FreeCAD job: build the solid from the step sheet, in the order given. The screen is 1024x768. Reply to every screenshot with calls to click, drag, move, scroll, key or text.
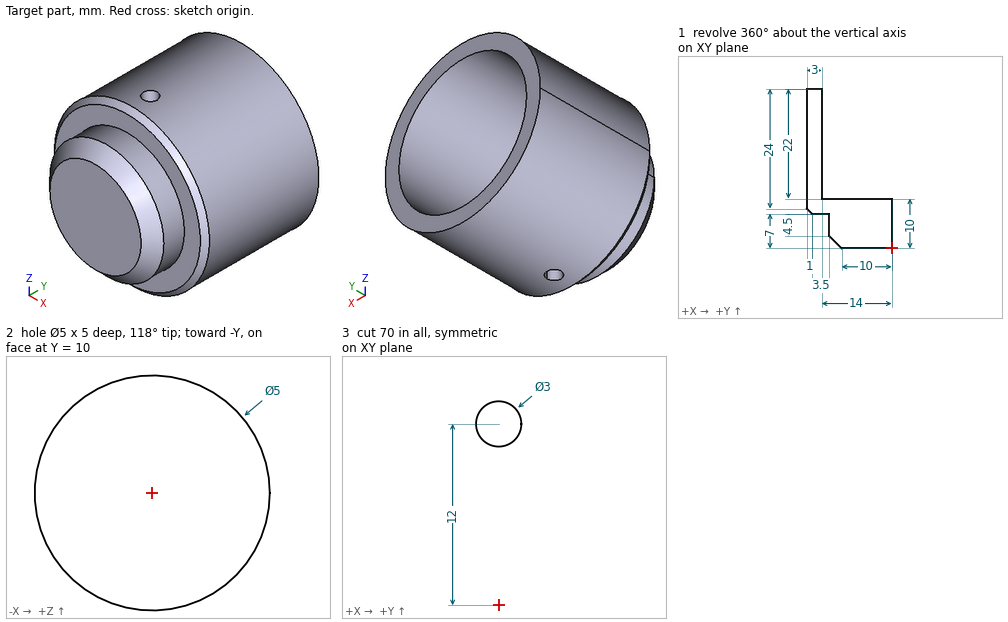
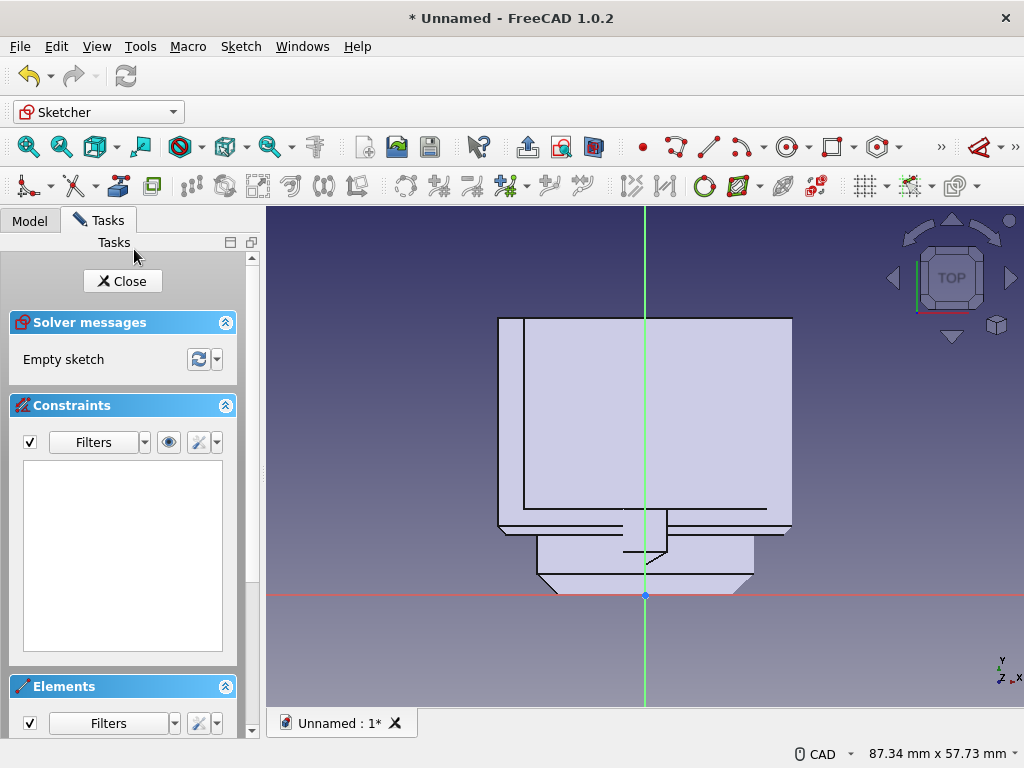
scroll(652, 495, up, 12)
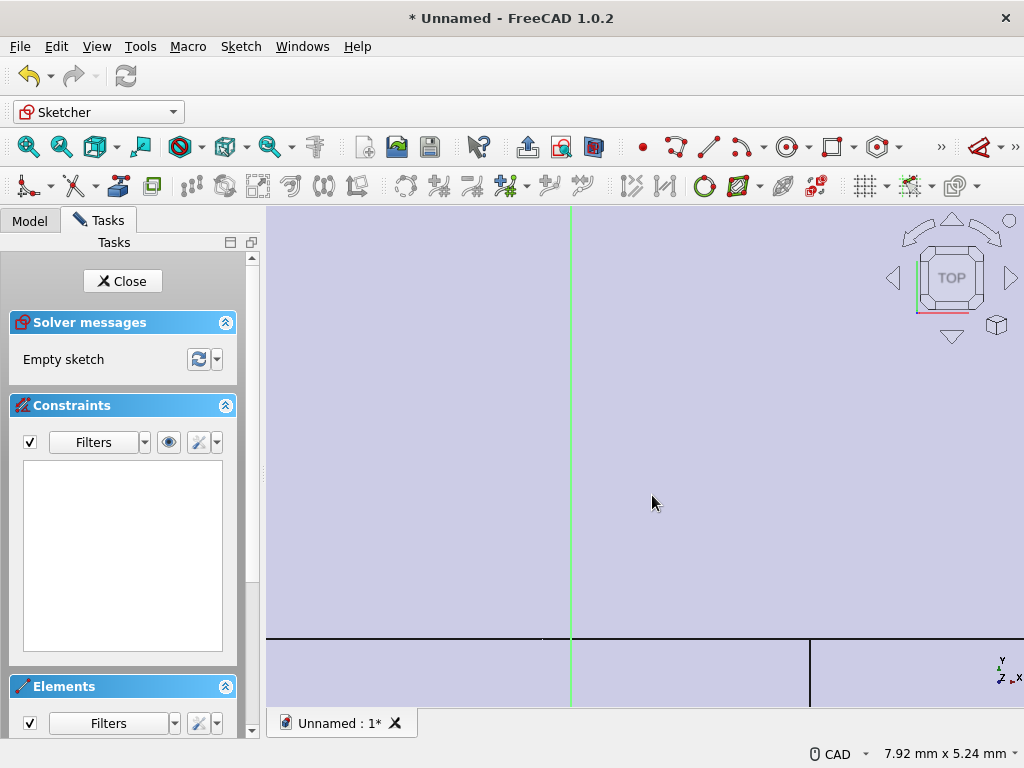
key(g)
key(c)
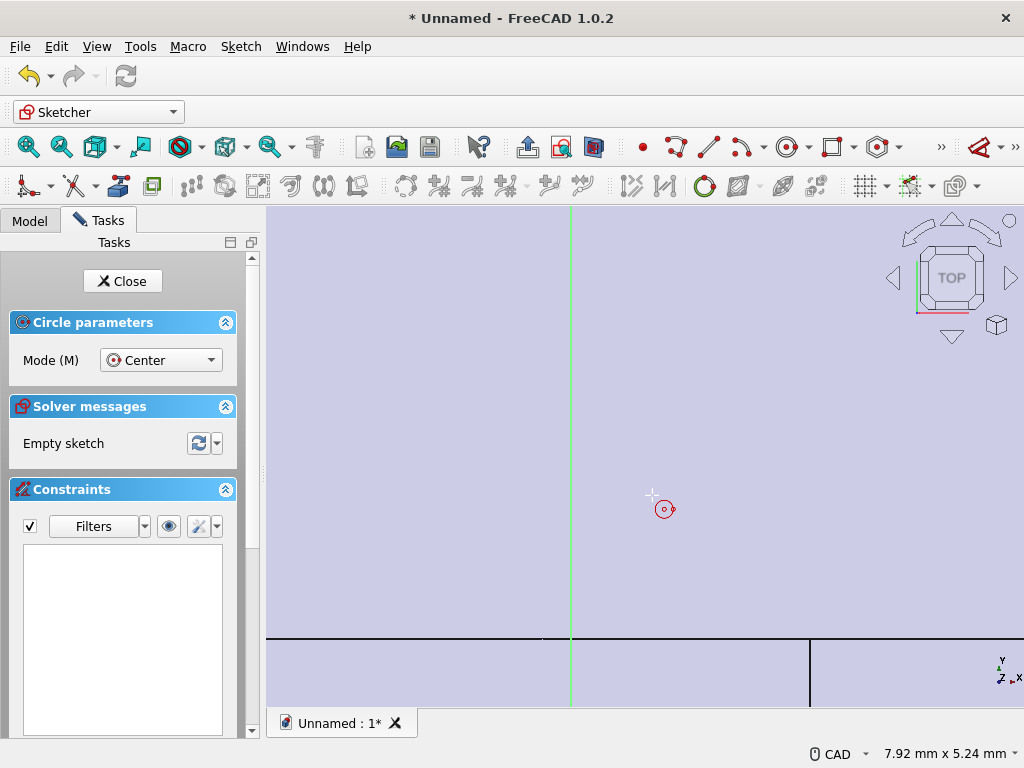
click(571, 447)
click(673, 346)
key(Escape)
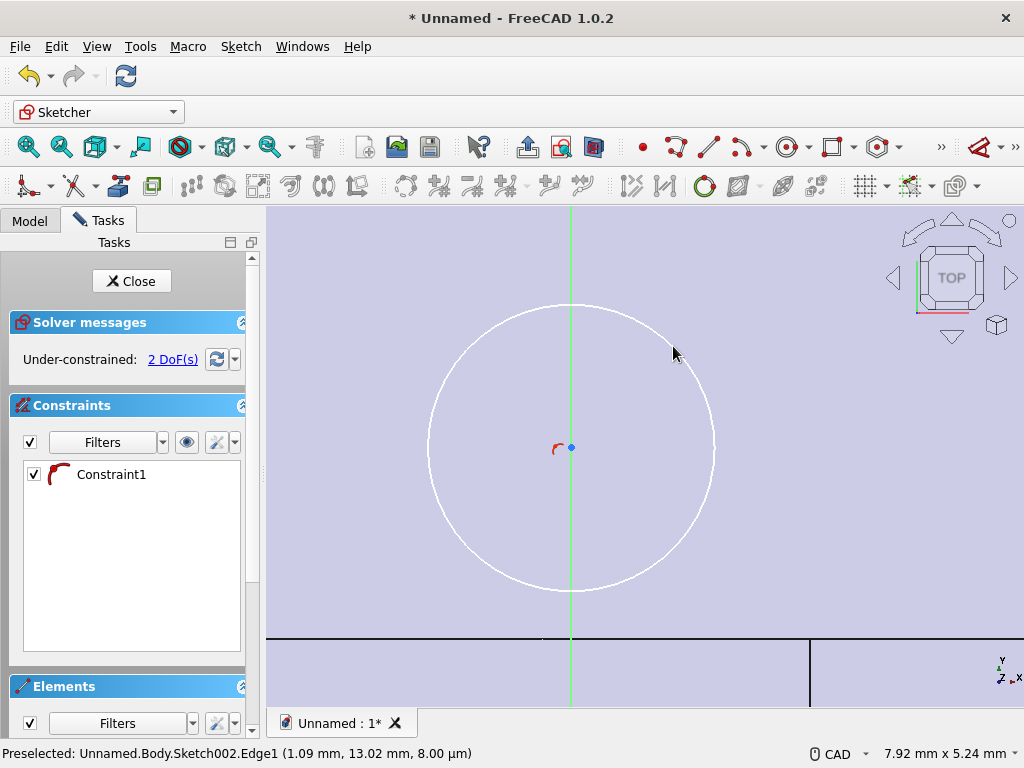
click(978, 148)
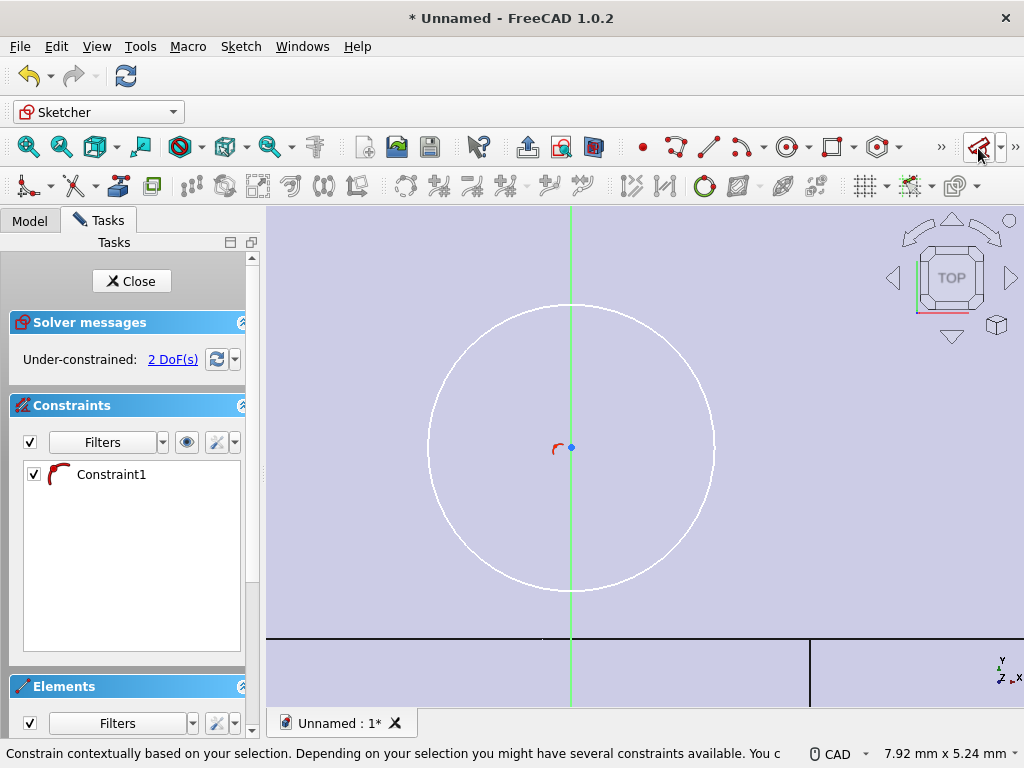
click(672, 346)
click(694, 323)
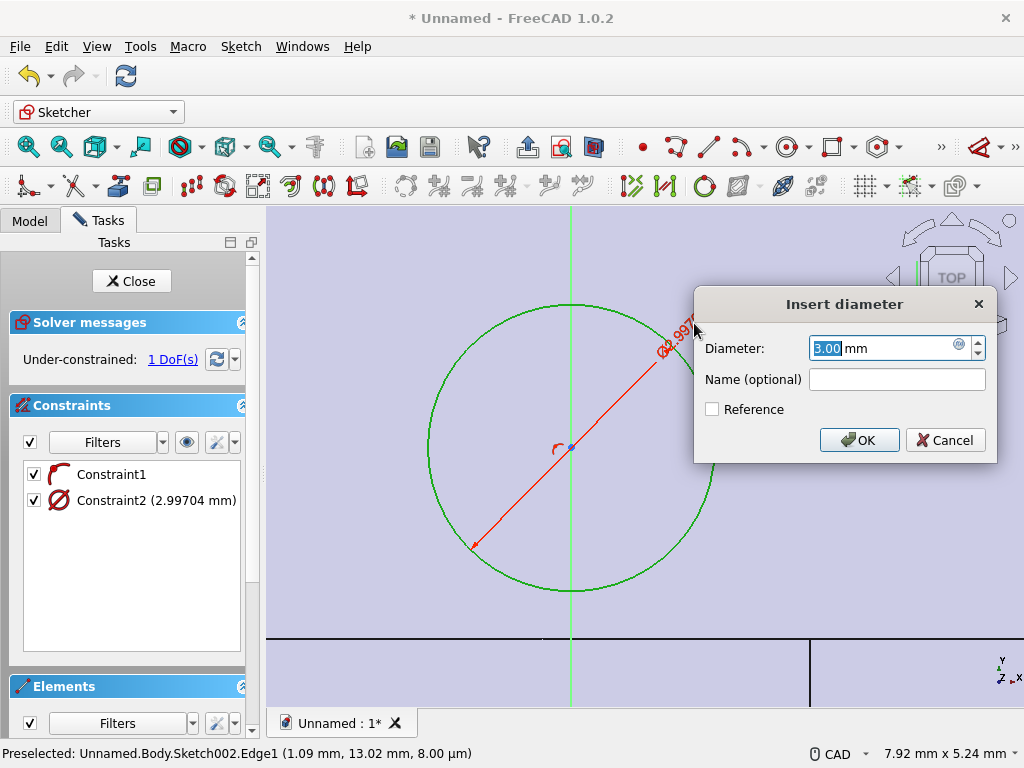
text(3)
key(Return)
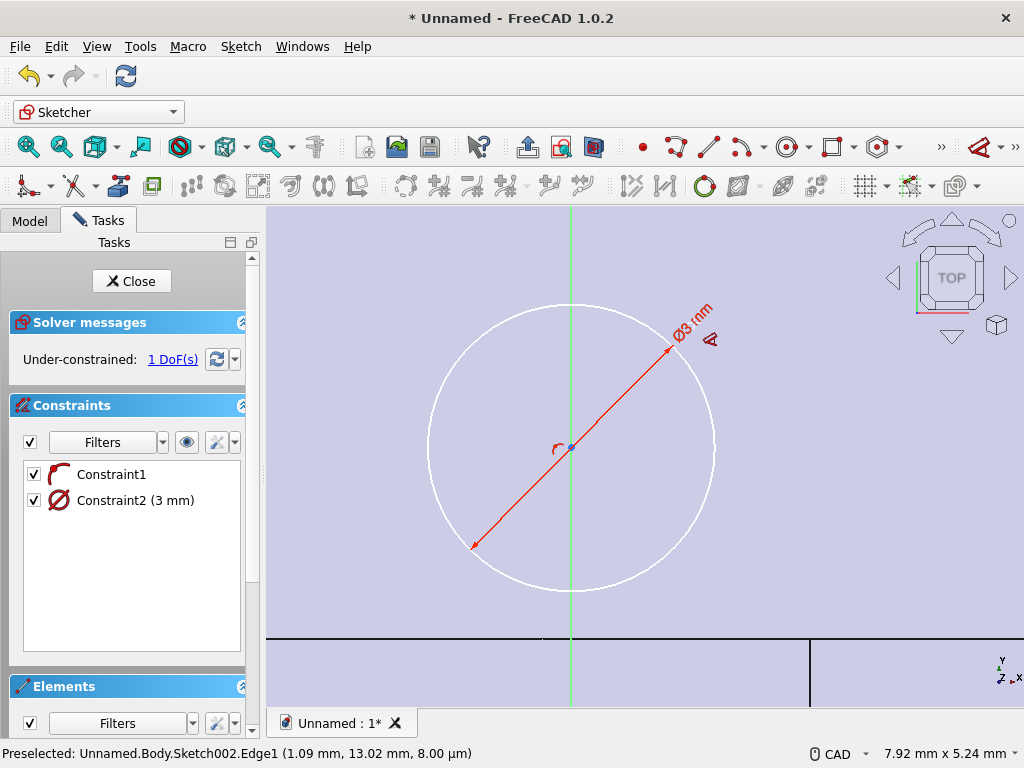
click(571, 448)
click(605, 563)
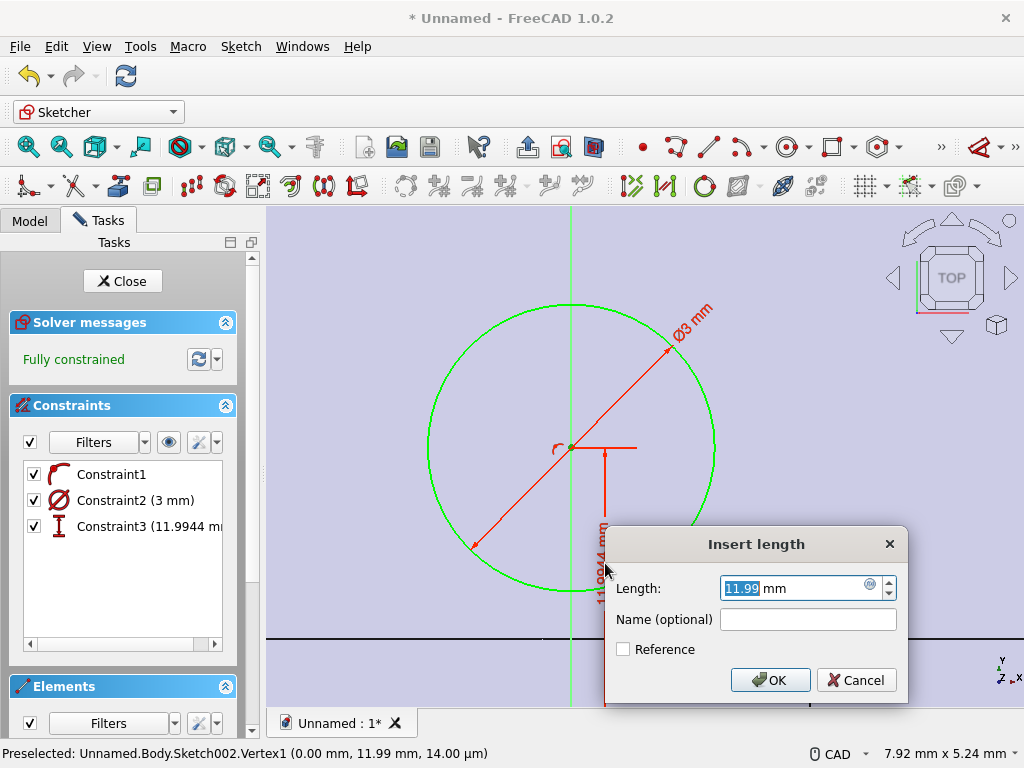
text(12)
key(Return)
key(Escape)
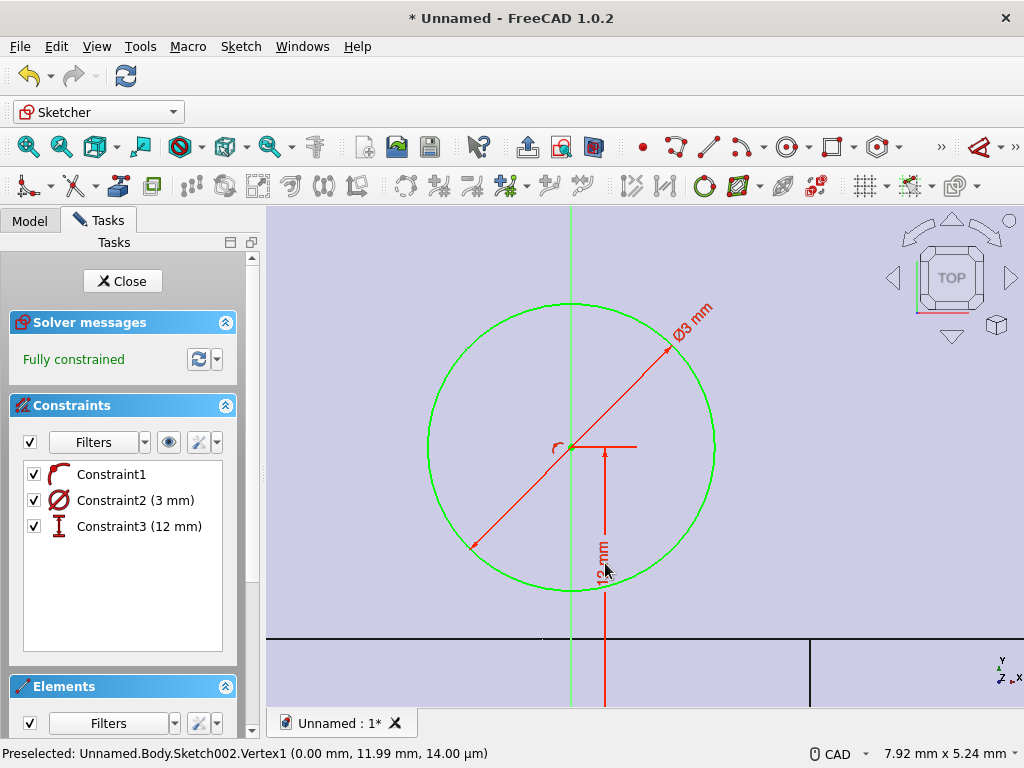
click(123, 281)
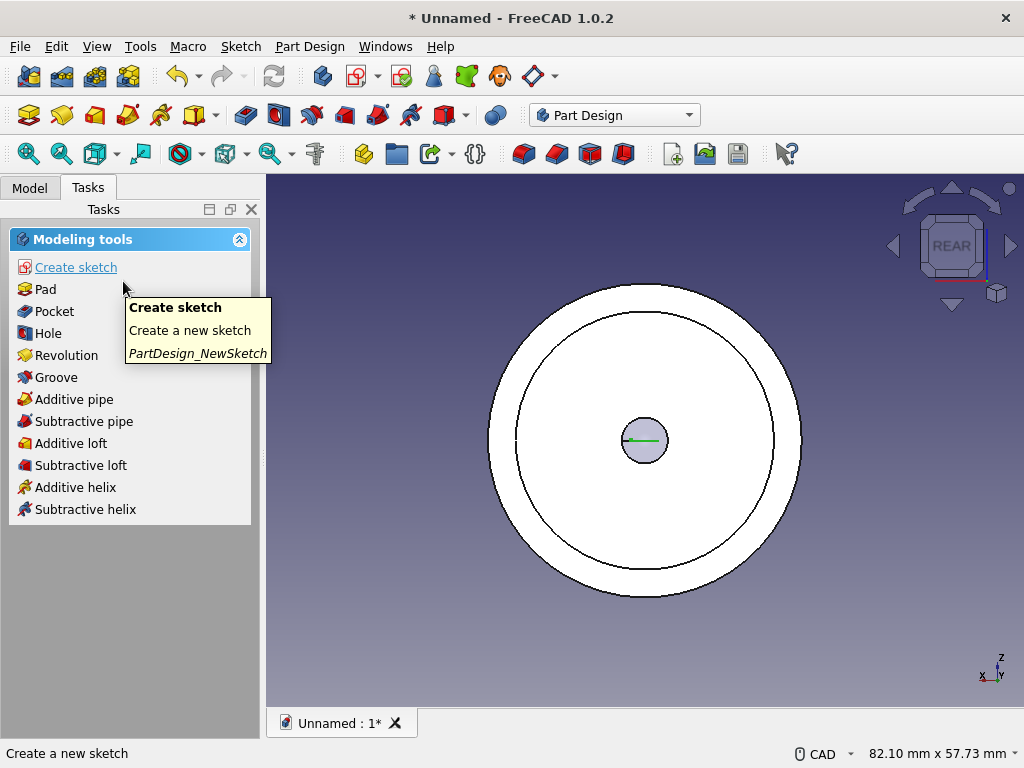
click(246, 116)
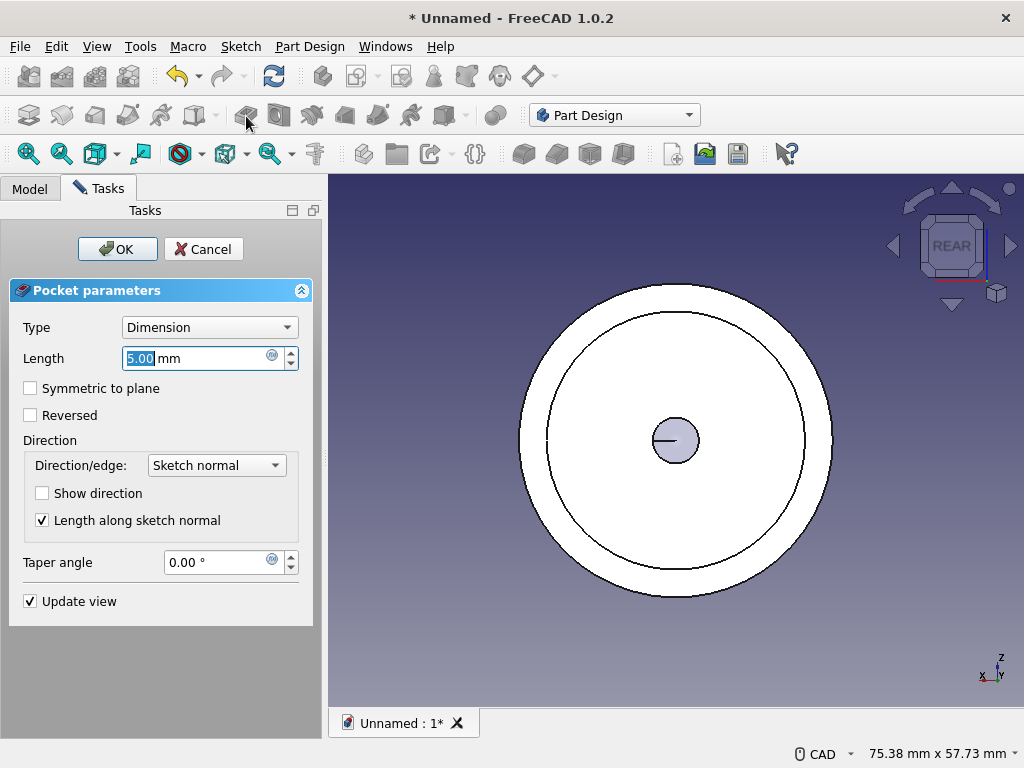
text(70)
key(Tab)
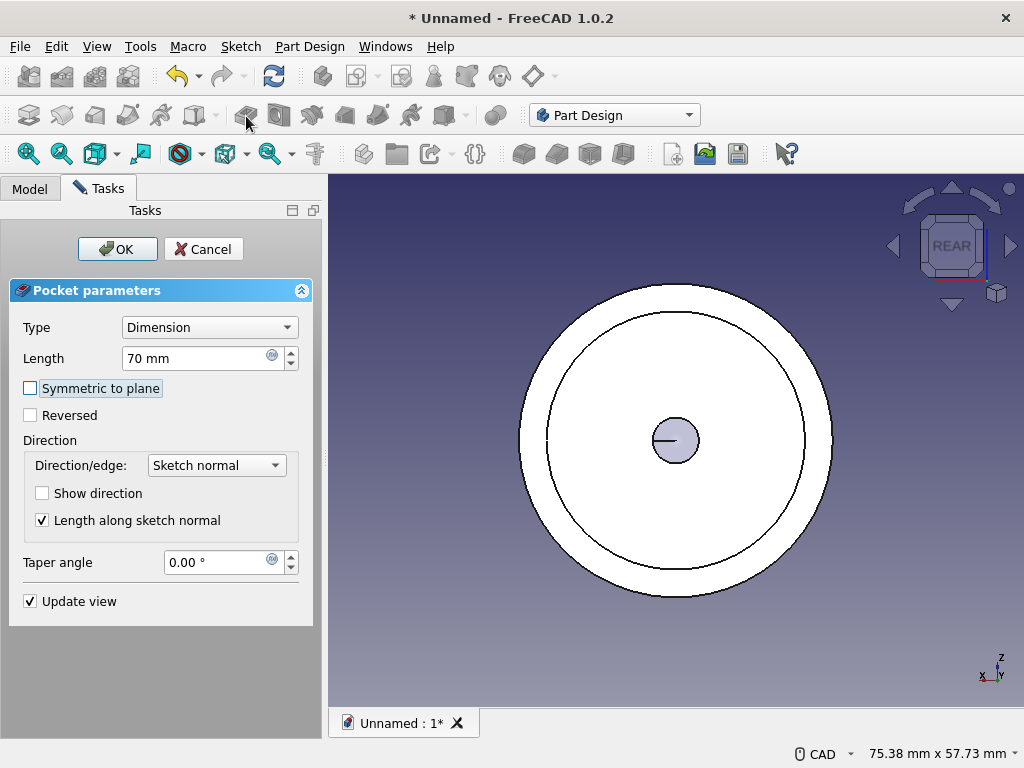
click(31, 388)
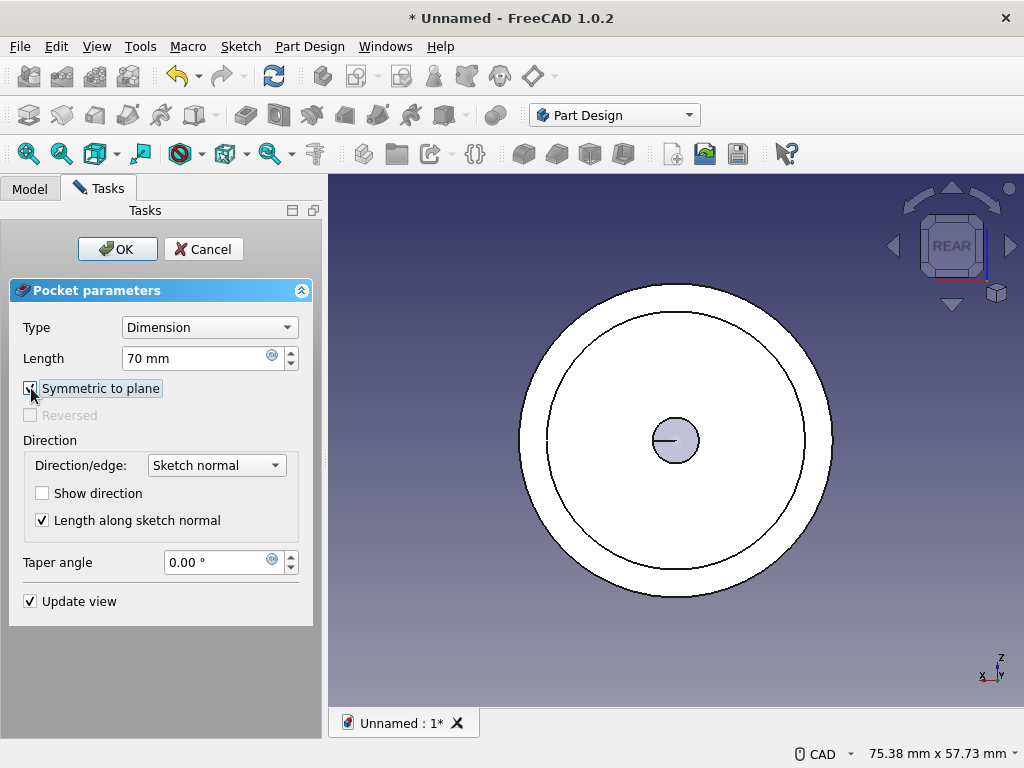
click(118, 249)